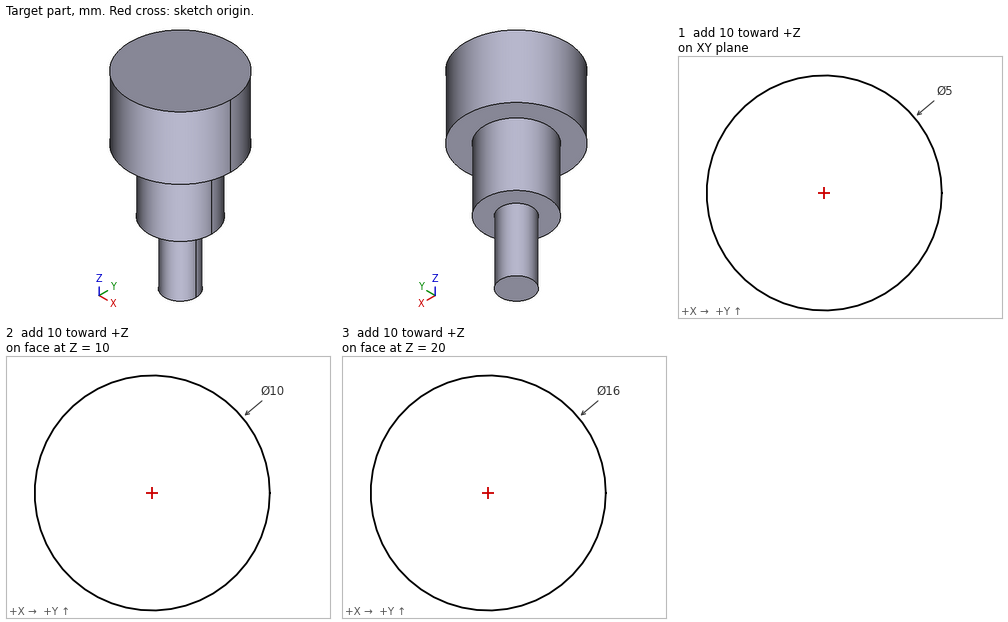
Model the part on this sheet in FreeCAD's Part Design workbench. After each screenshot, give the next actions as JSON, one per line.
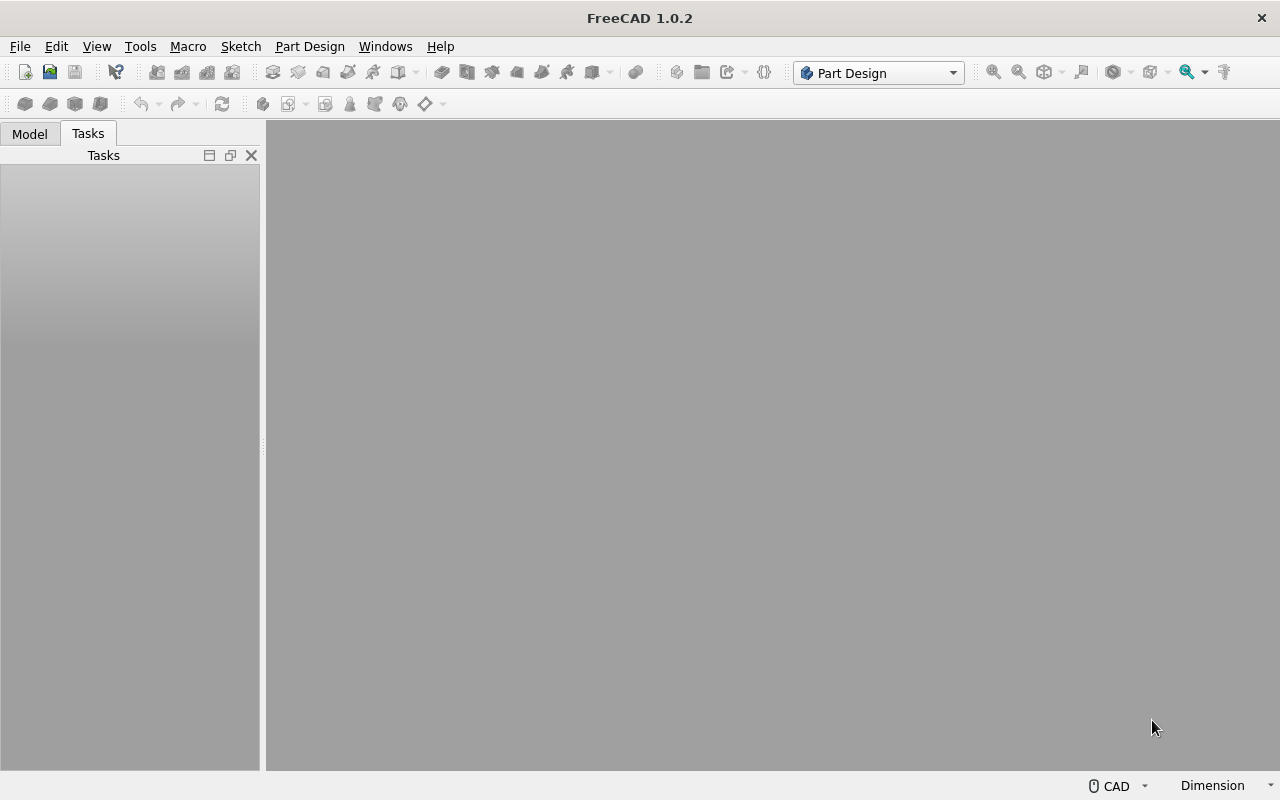
{"action": "left_click", "coordinate": [25, 72]}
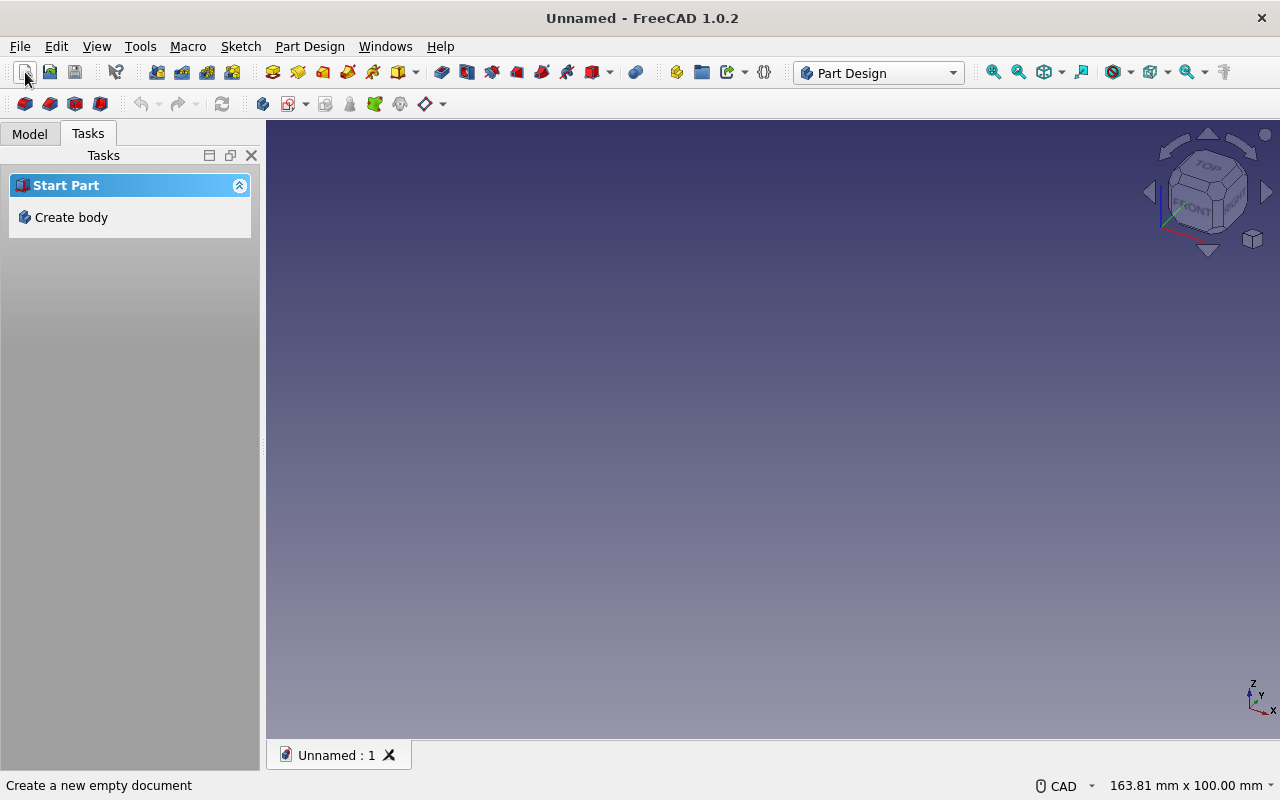
{"action": "left_click", "coordinate": [288, 104]}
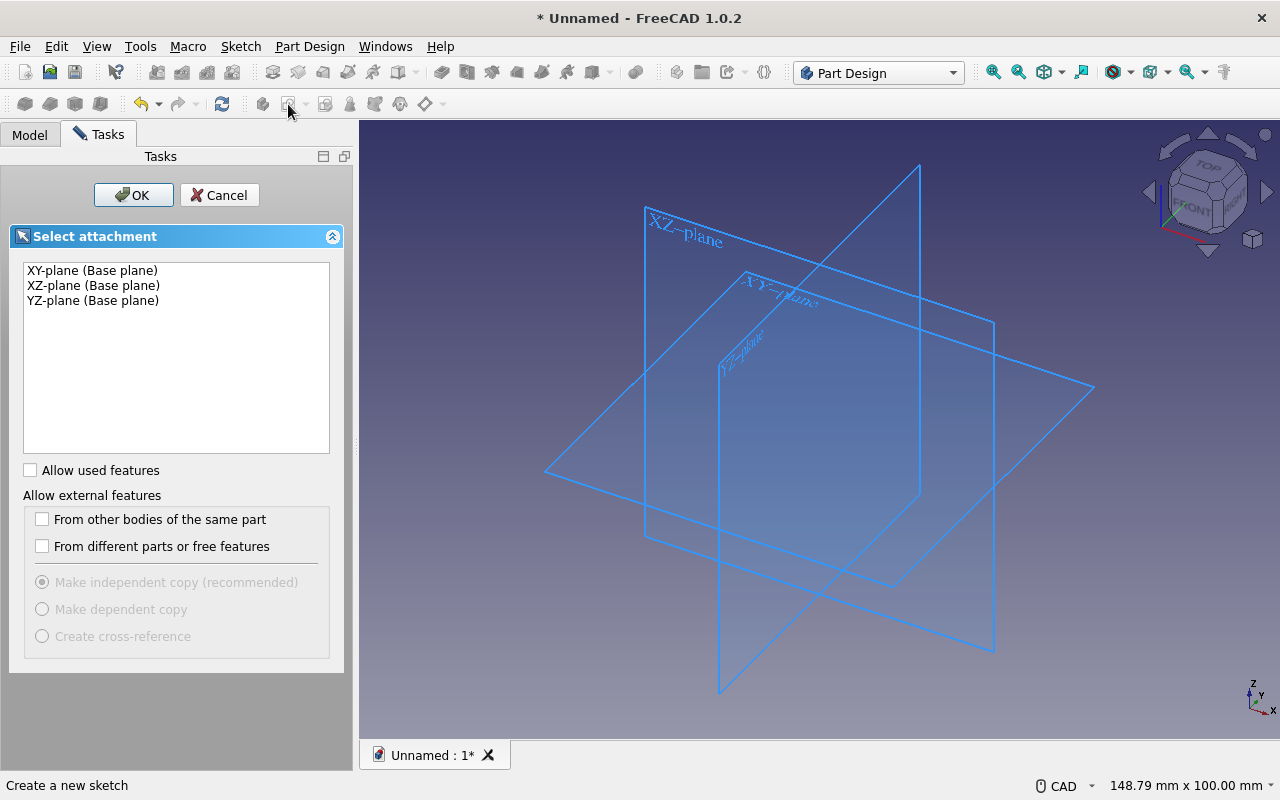
{"action": "left_click", "coordinate": [84, 270]}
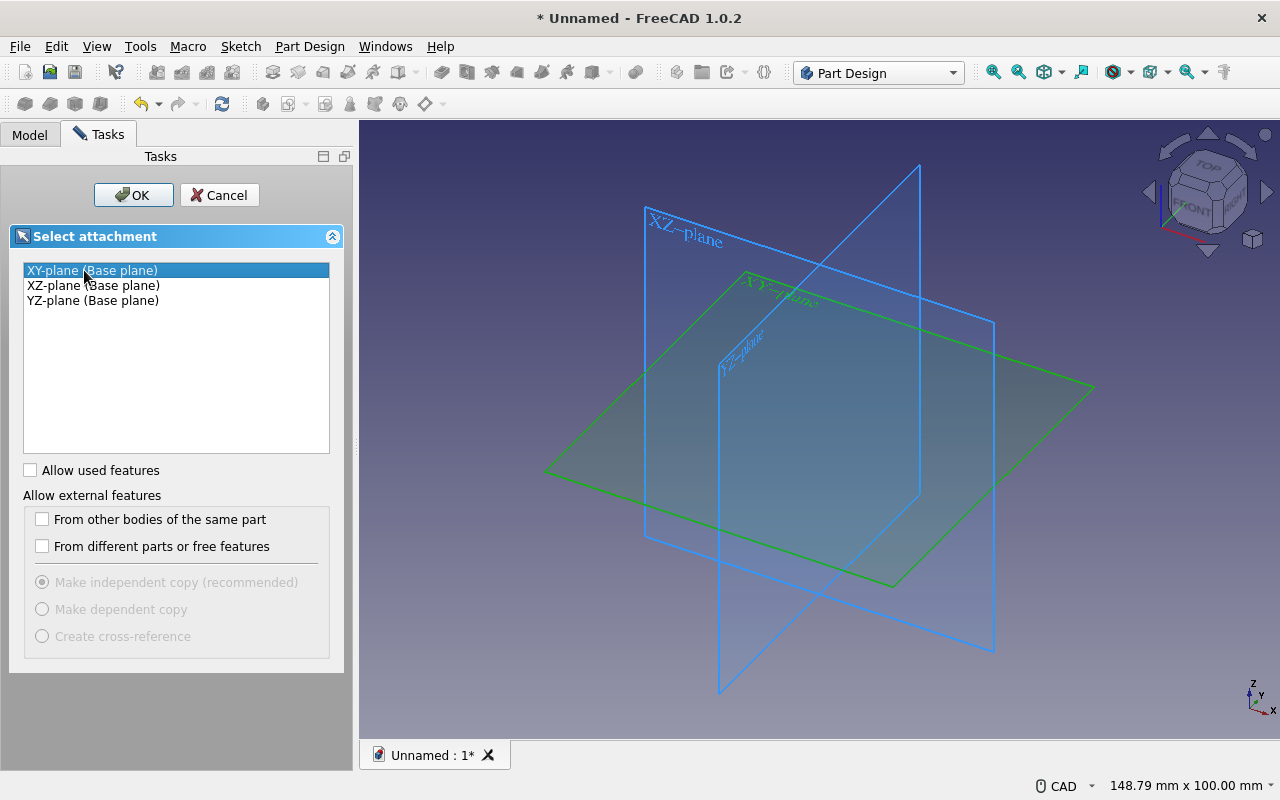
{"action": "left_click", "coordinate": [134, 195]}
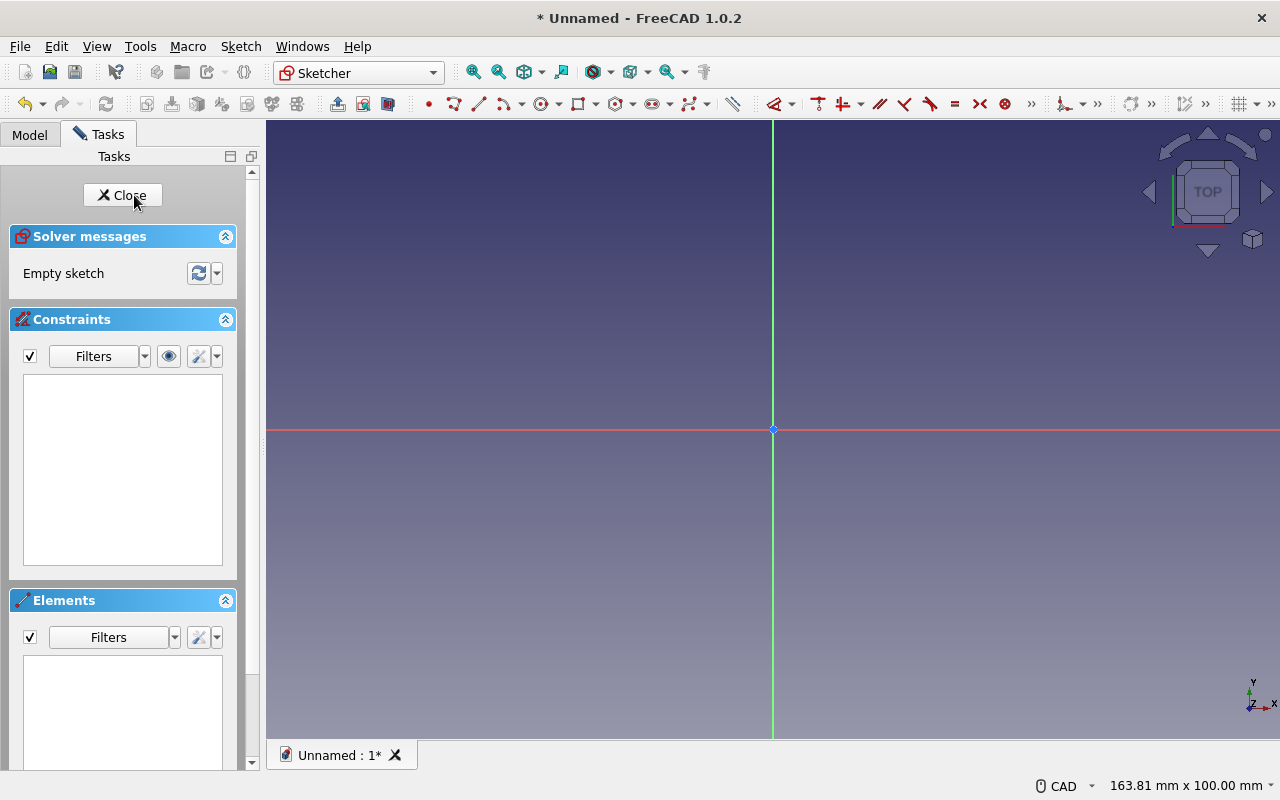
{"action": "scroll", "coordinate": [778, 430], "scroll_direction": "up", "scroll_amount": 13}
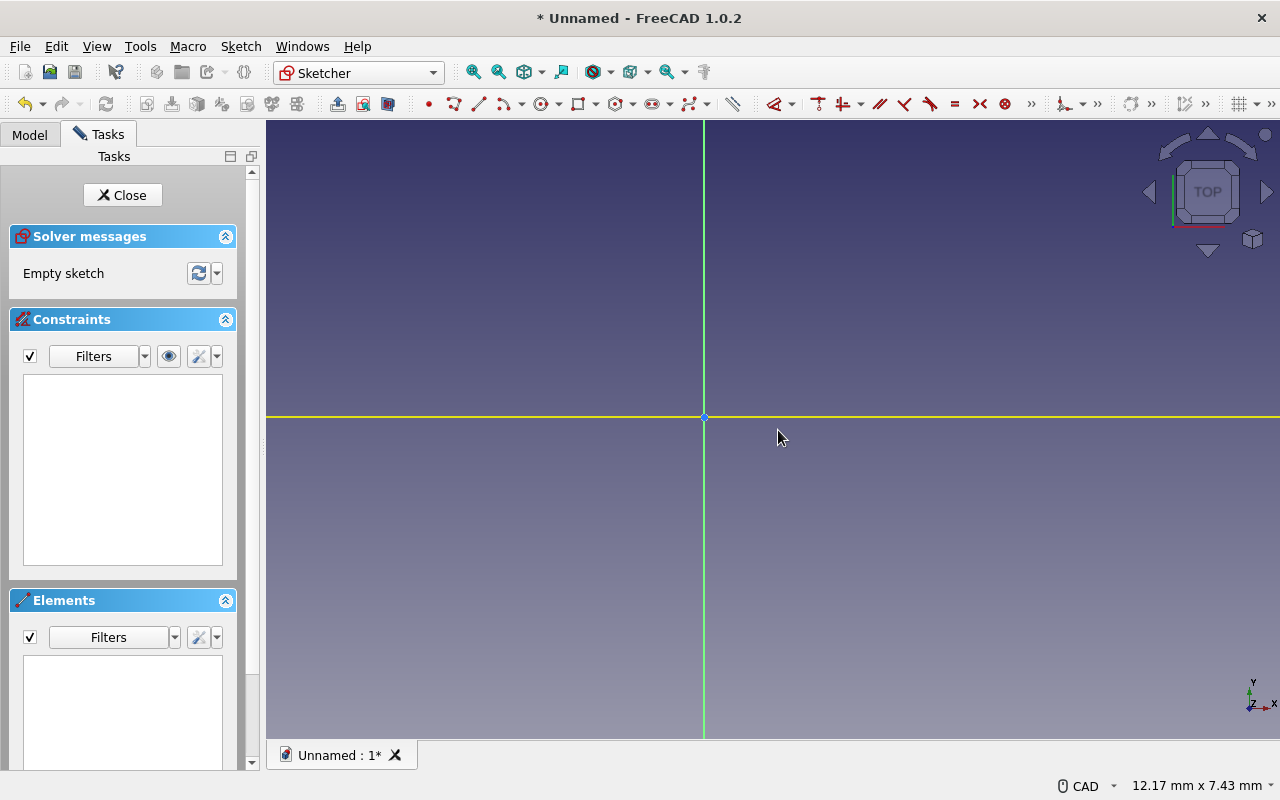
{"action": "left_click", "coordinate": [540, 104]}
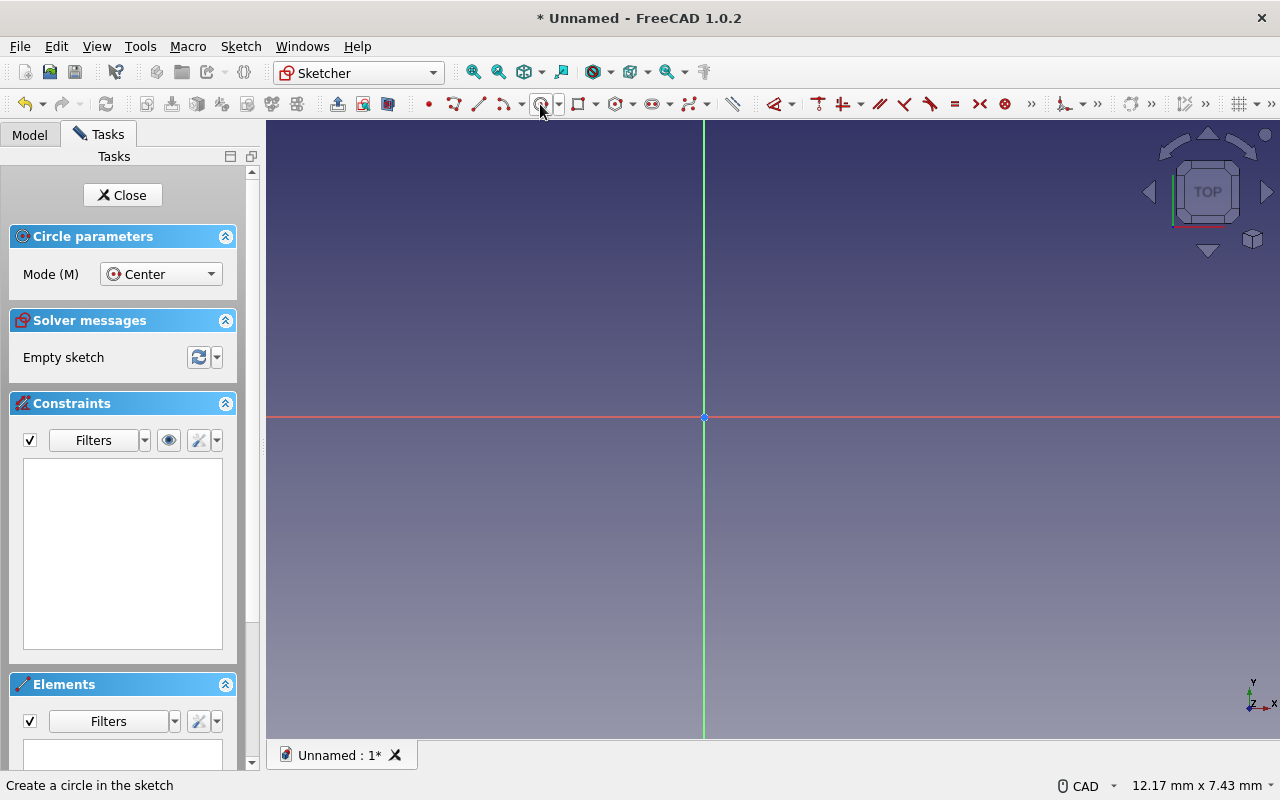
{"action": "left_click", "coordinate": [704, 417]}
{"action": "left_click", "coordinate": [852, 270]}
{"action": "key", "text": "Escape"}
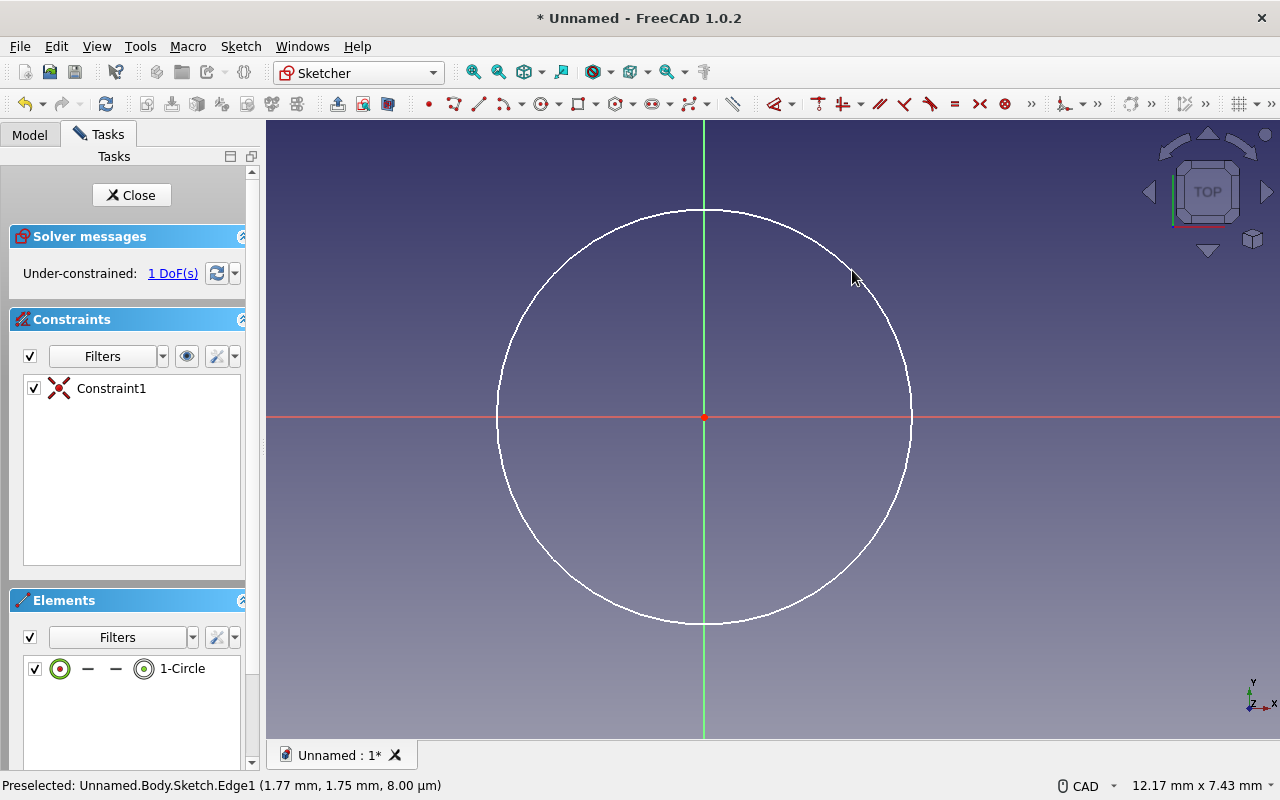
{"action": "left_click", "coordinate": [774, 104]}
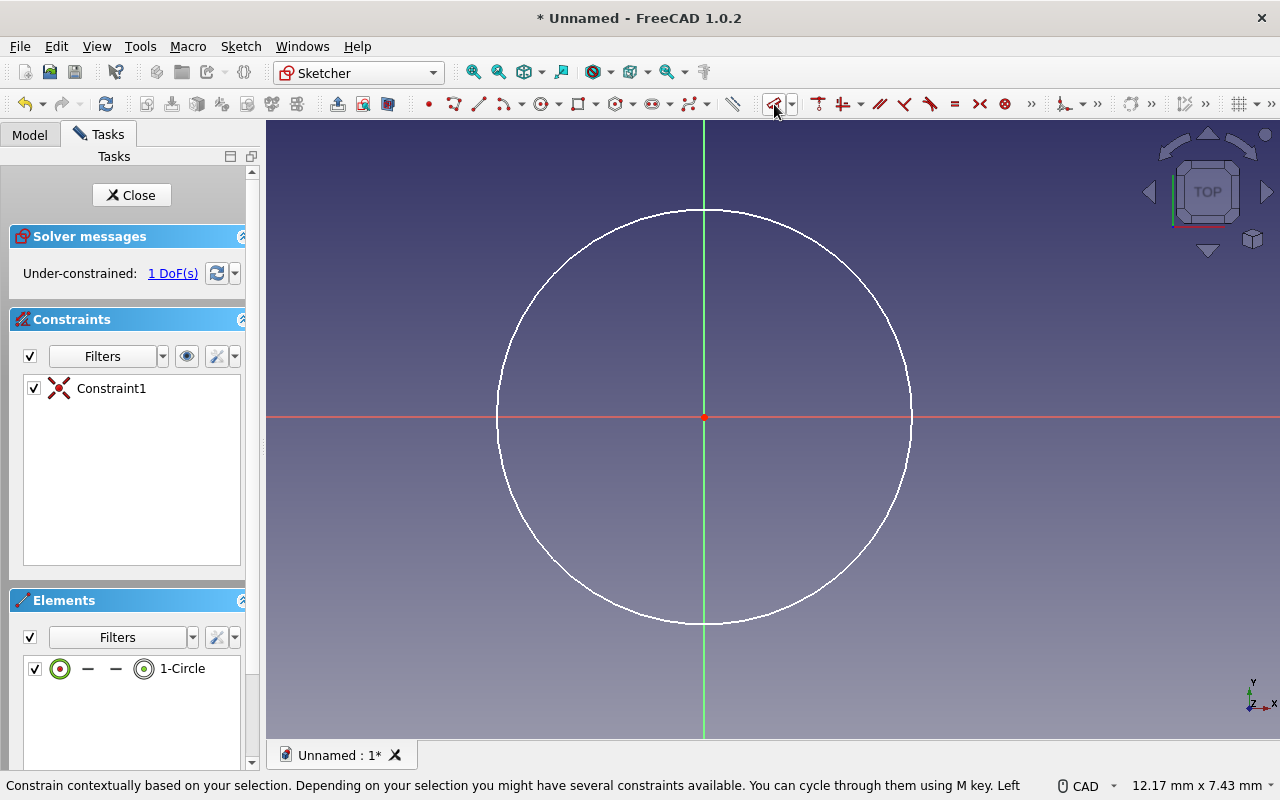
{"action": "left_click", "coordinate": [851, 270]}
{"action": "left_click", "coordinate": [874, 247]}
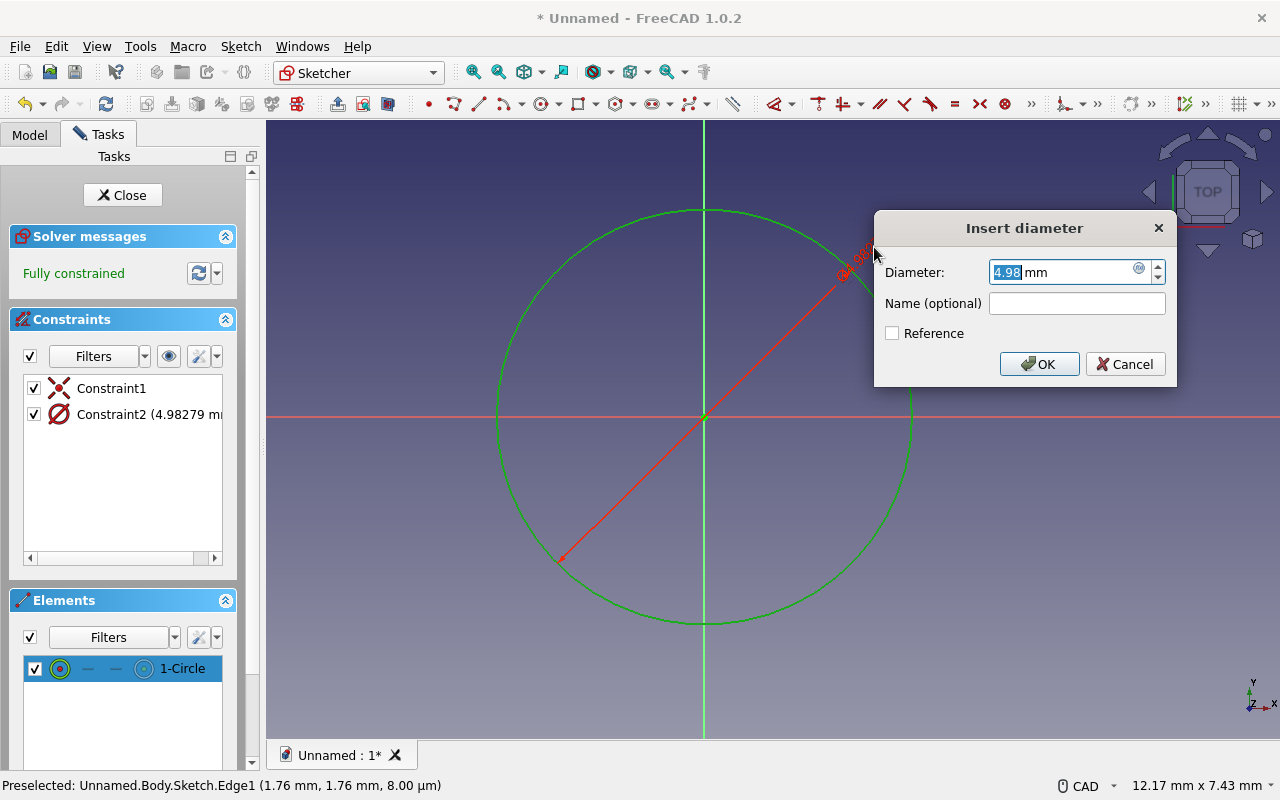
{"action": "type", "text": "5"}
{"action": "key", "text": "Return"}
{"action": "key", "text": "Escape"}